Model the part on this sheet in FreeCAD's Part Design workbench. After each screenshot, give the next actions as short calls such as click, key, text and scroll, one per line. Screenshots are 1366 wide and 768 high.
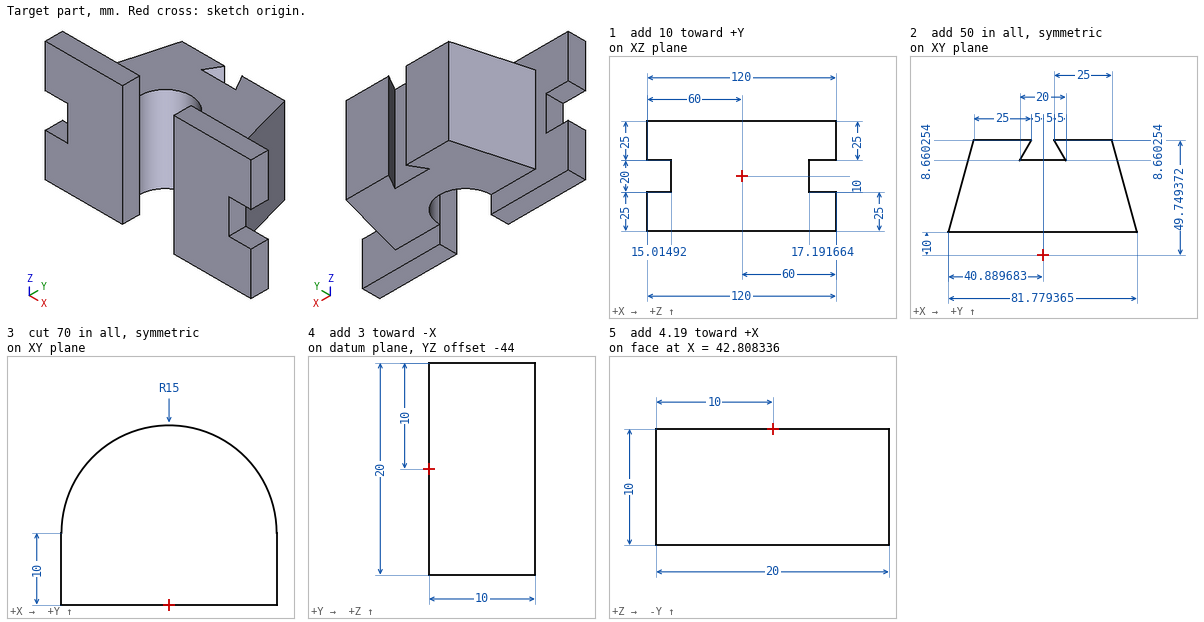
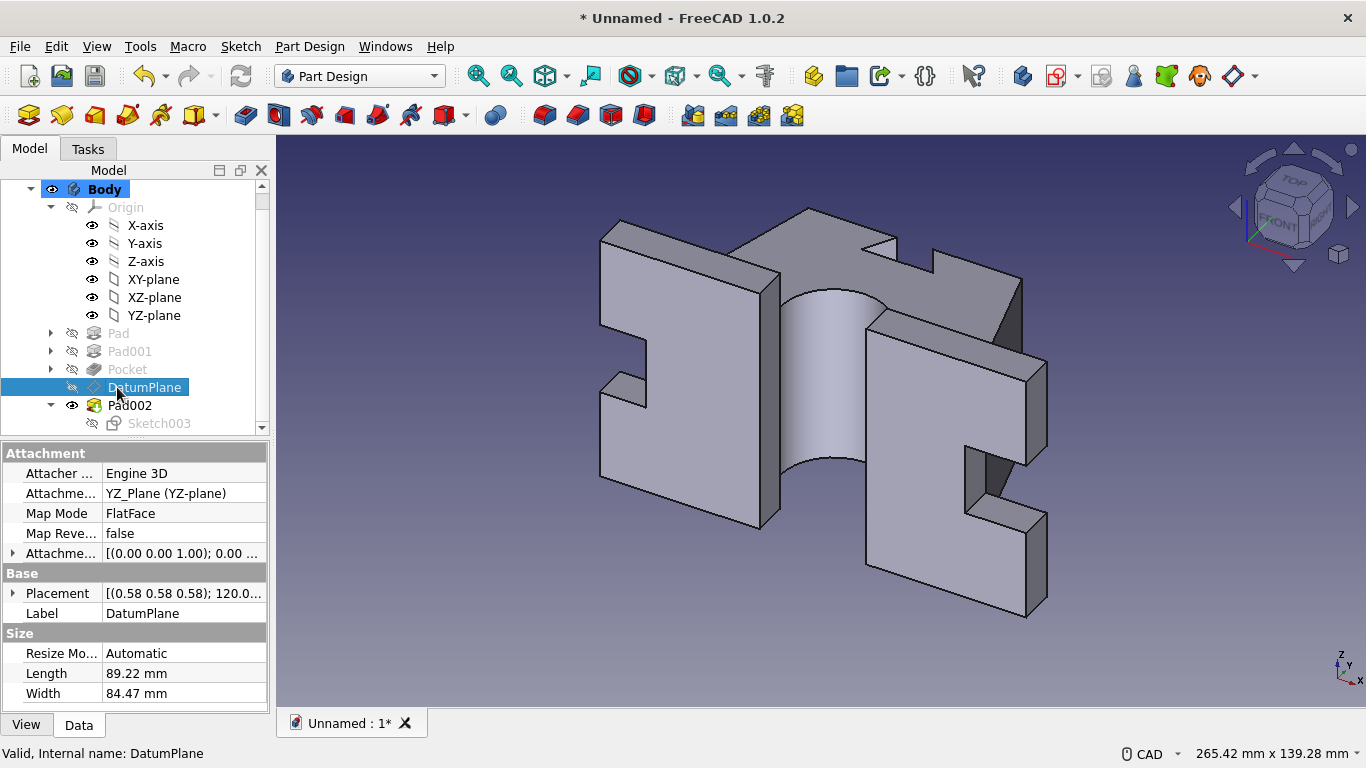
click(975, 468)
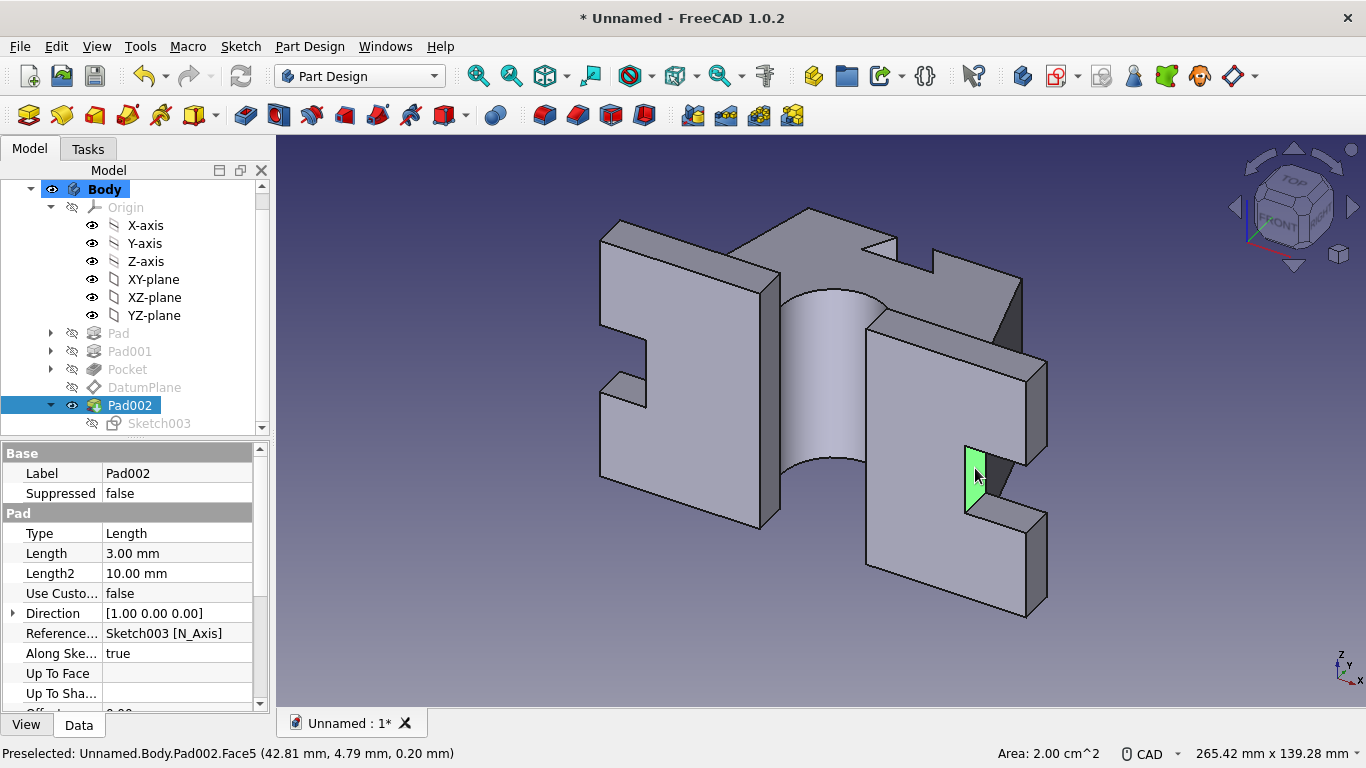
click(1056, 76)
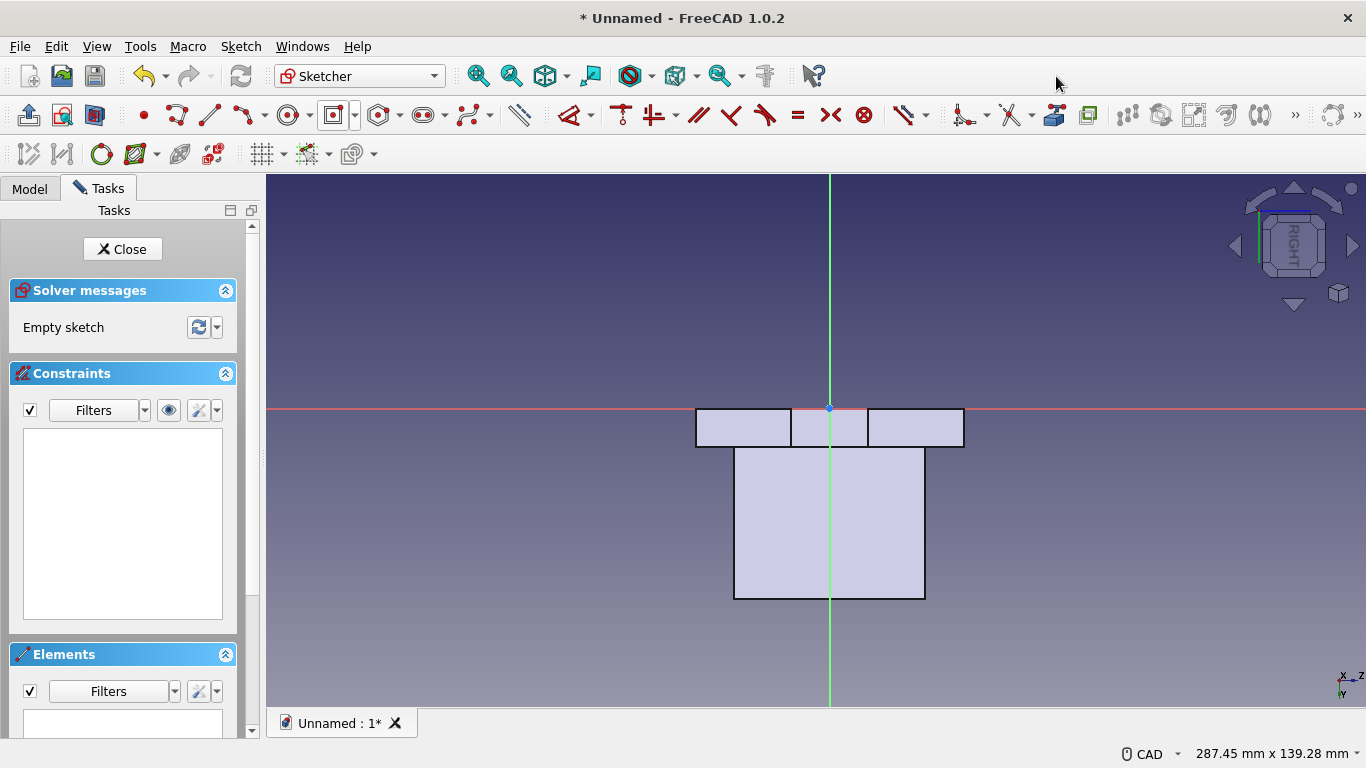
scroll(840, 426, up, 11)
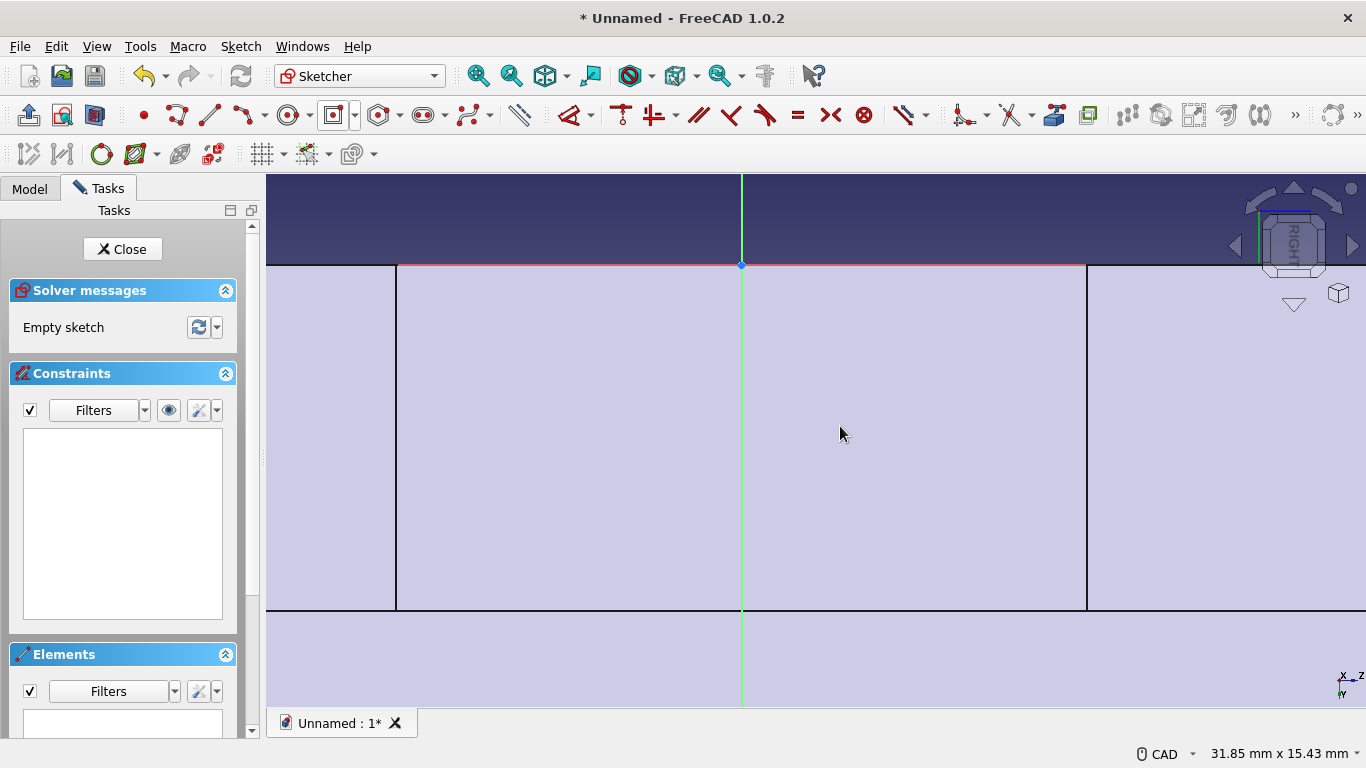
key(g)
key(r)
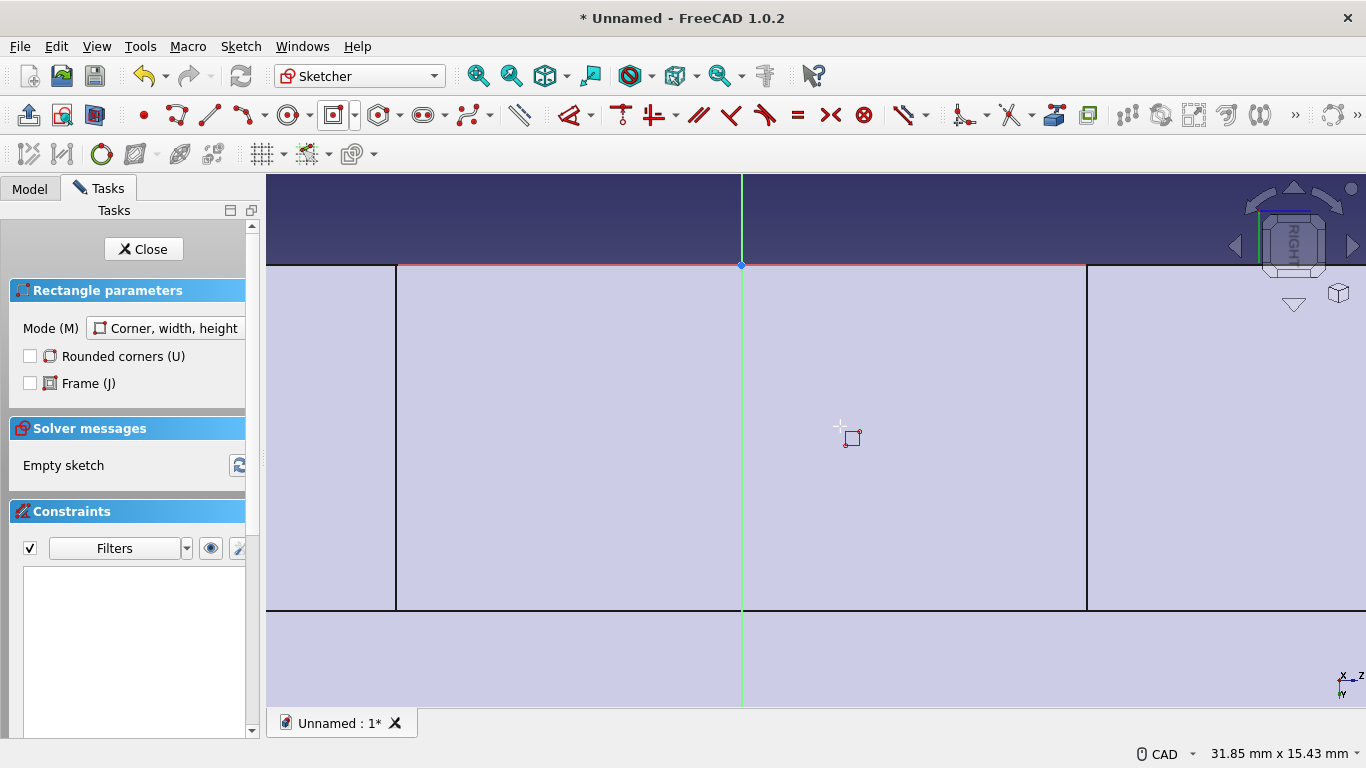
click(396, 265)
click(1087, 611)
key(Escape)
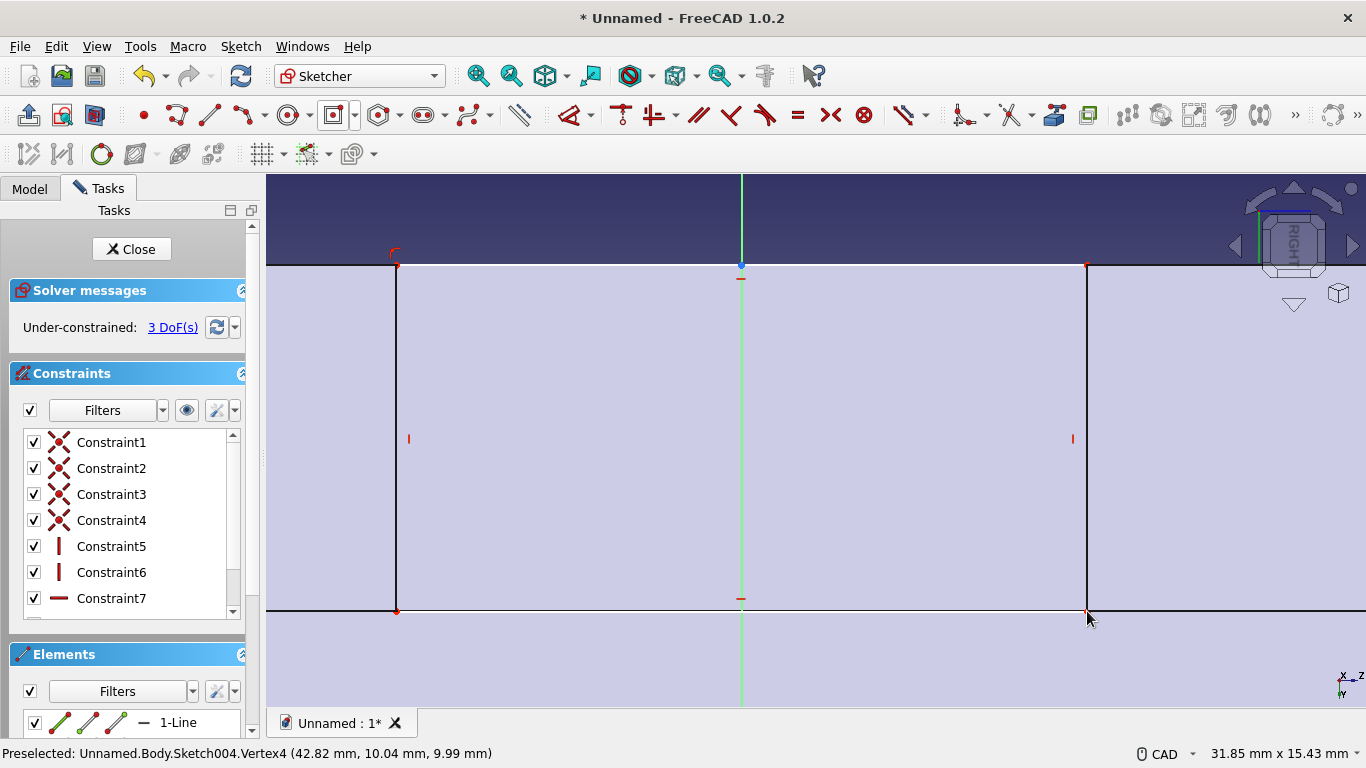
click(568, 116)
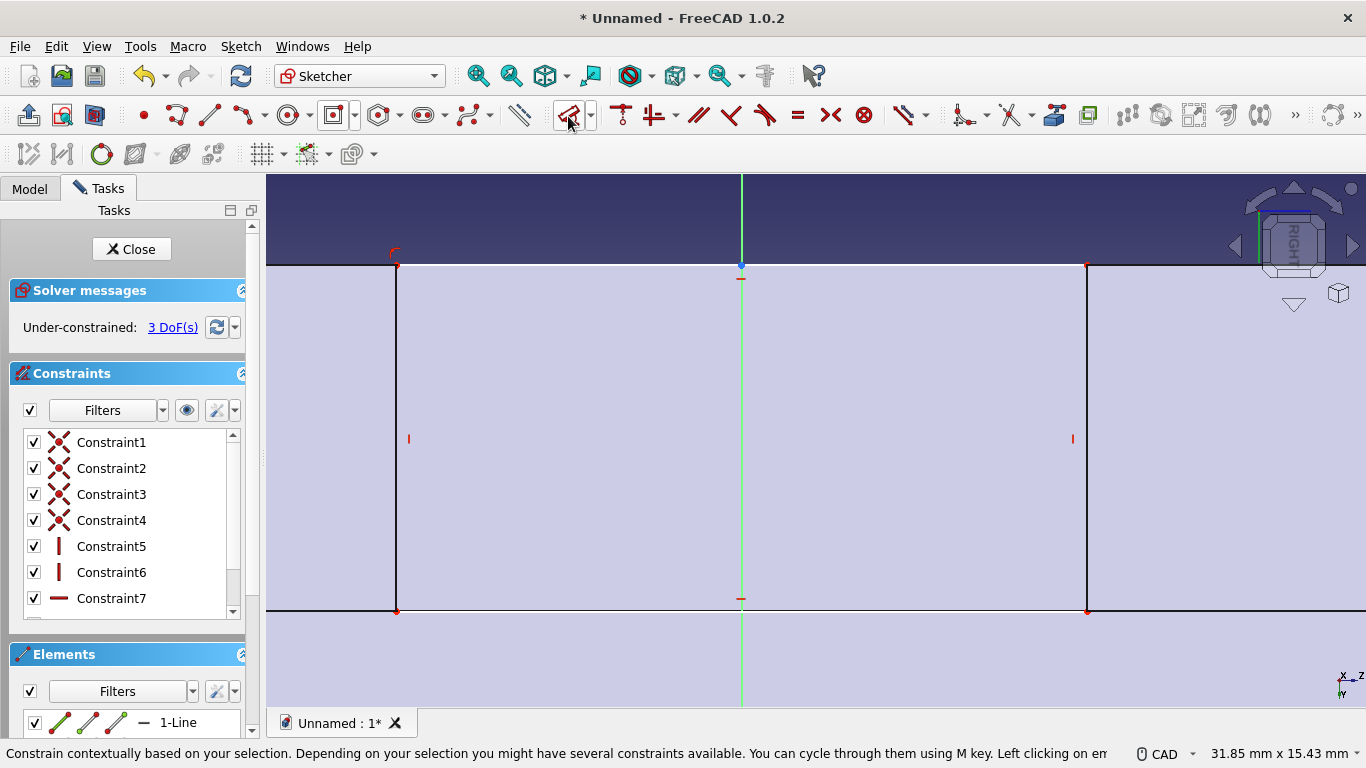
click(396, 369)
click(362, 439)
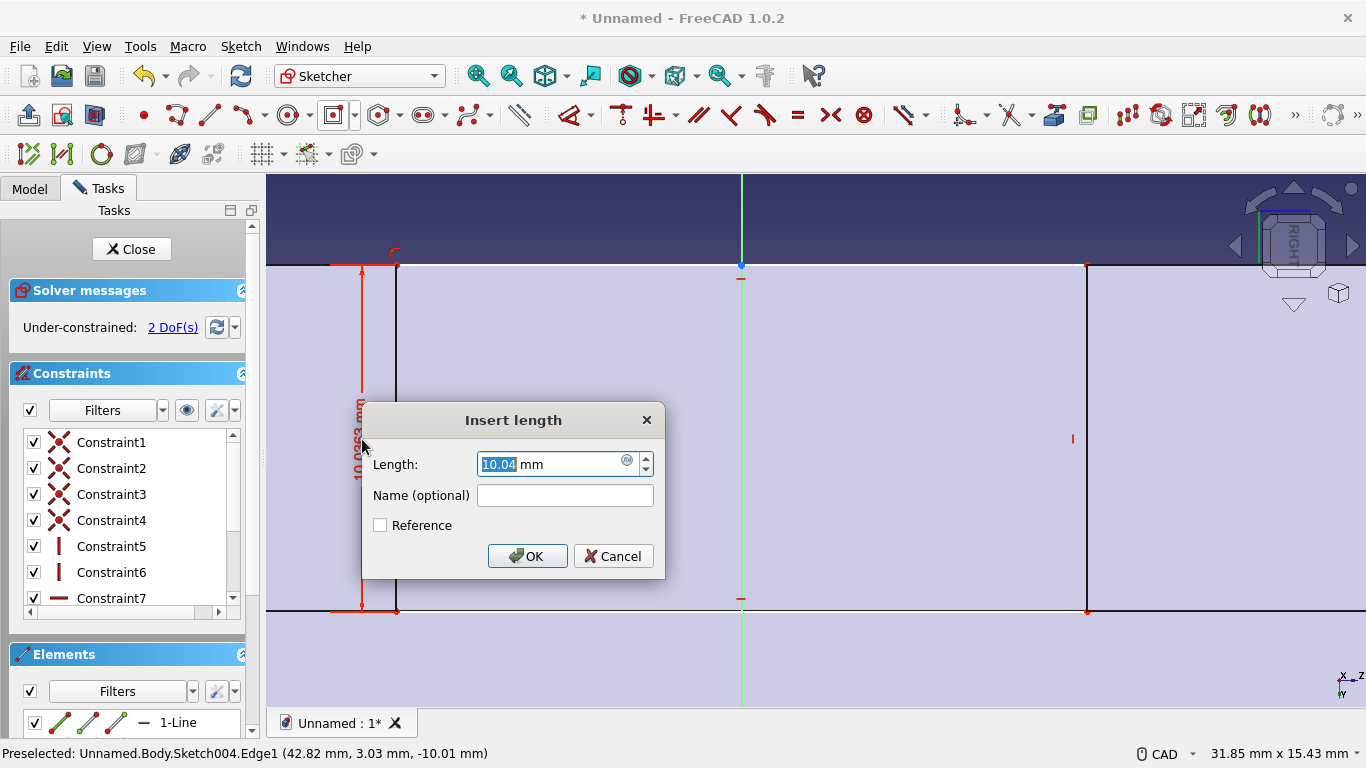
text(10)
key(Return)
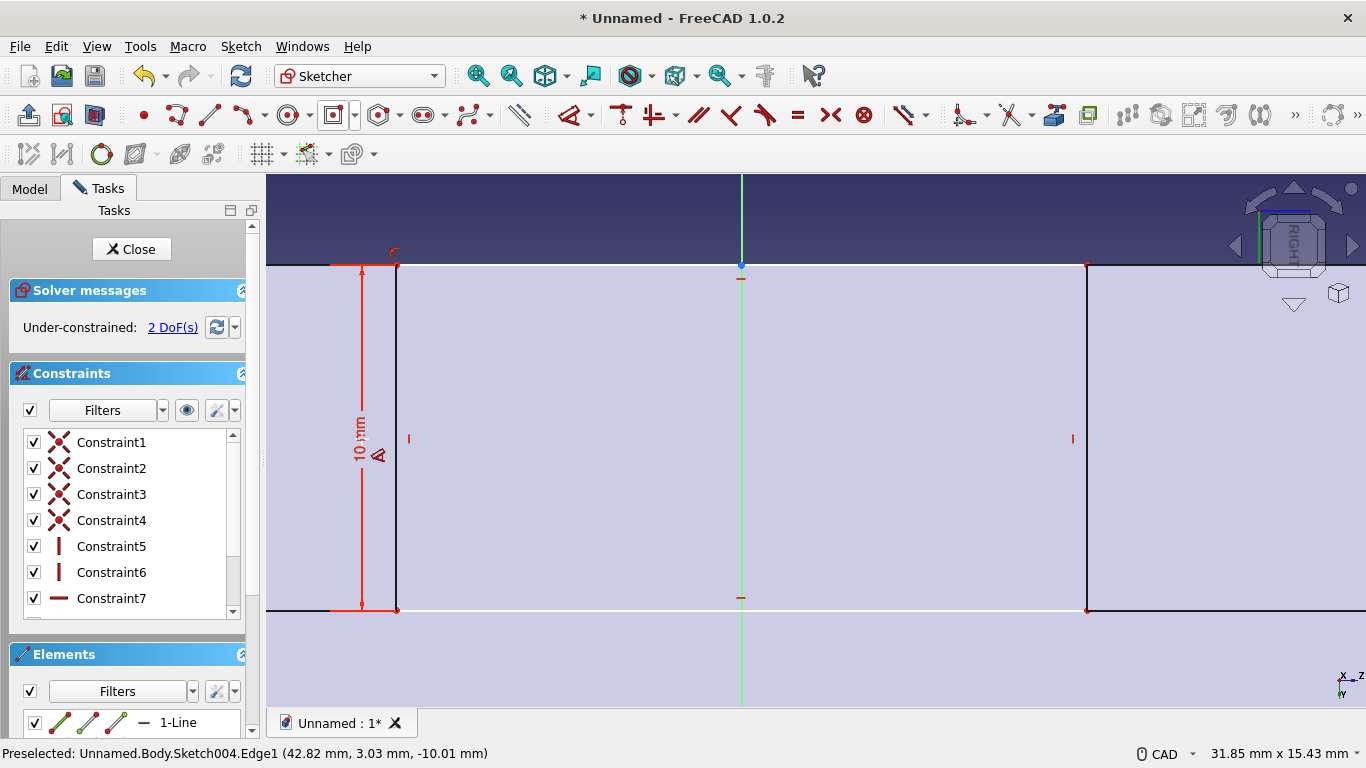
click(603, 611)
click(583, 645)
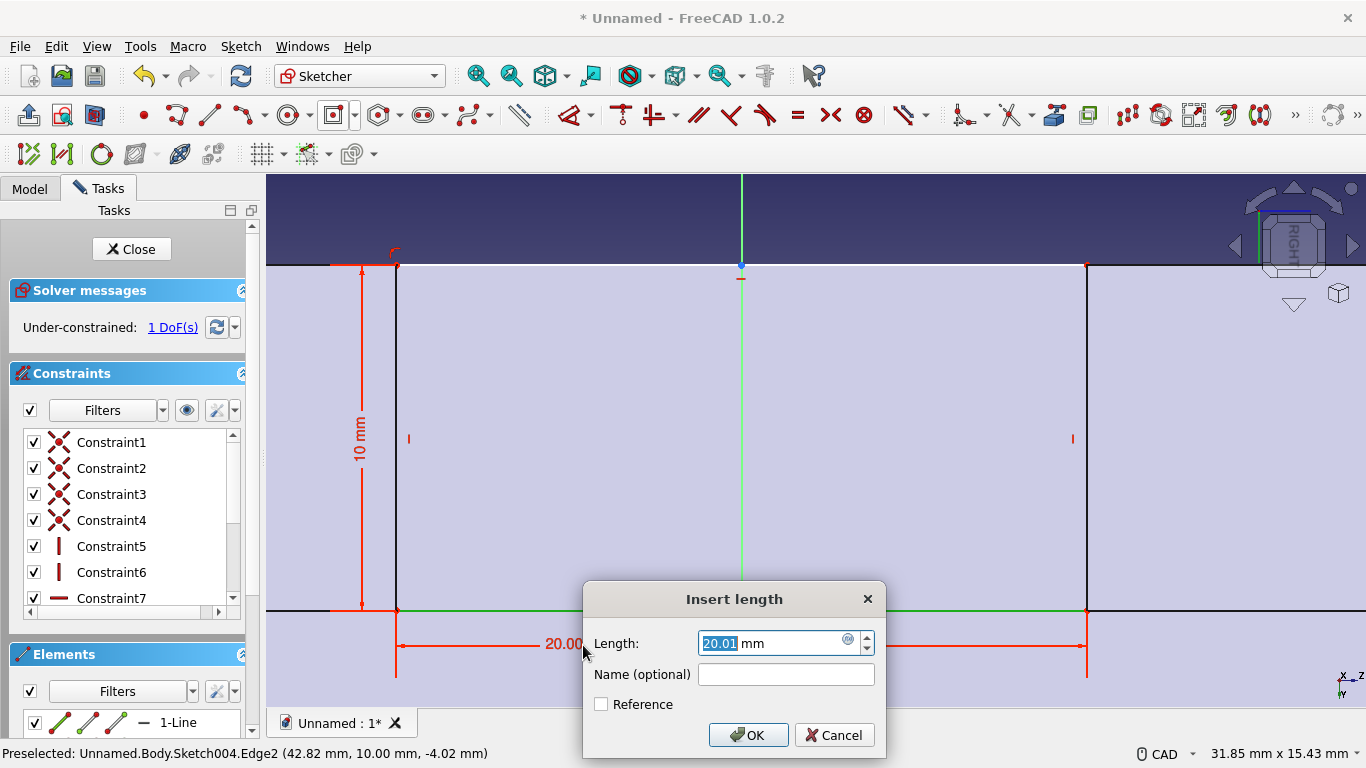
text(20)
key(Return)